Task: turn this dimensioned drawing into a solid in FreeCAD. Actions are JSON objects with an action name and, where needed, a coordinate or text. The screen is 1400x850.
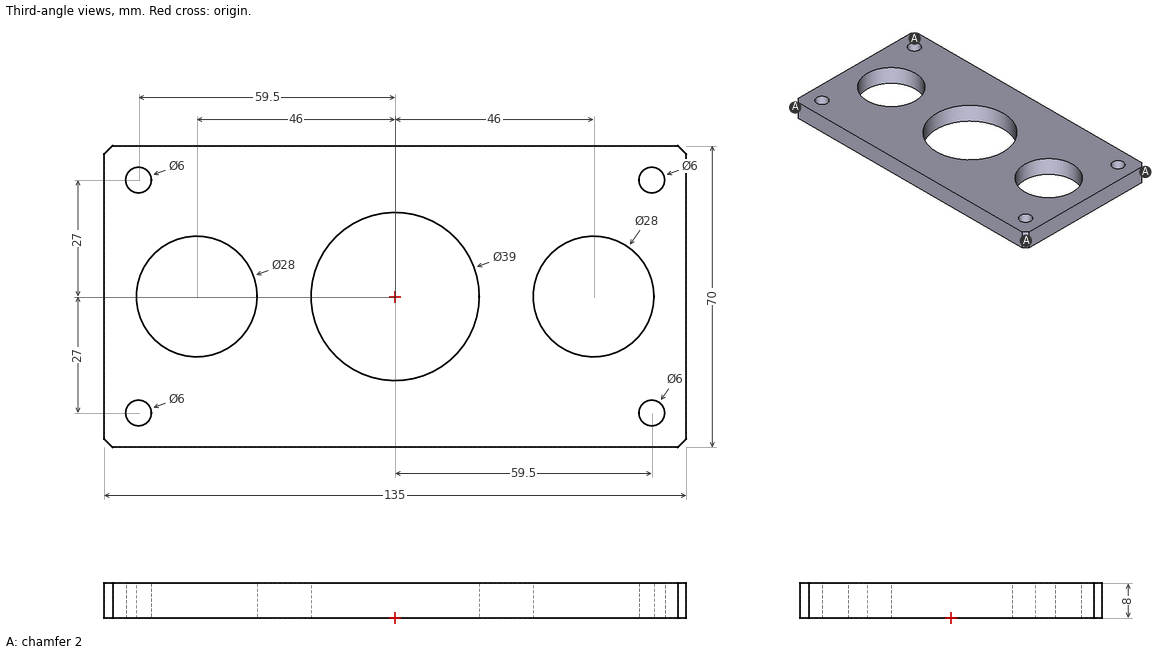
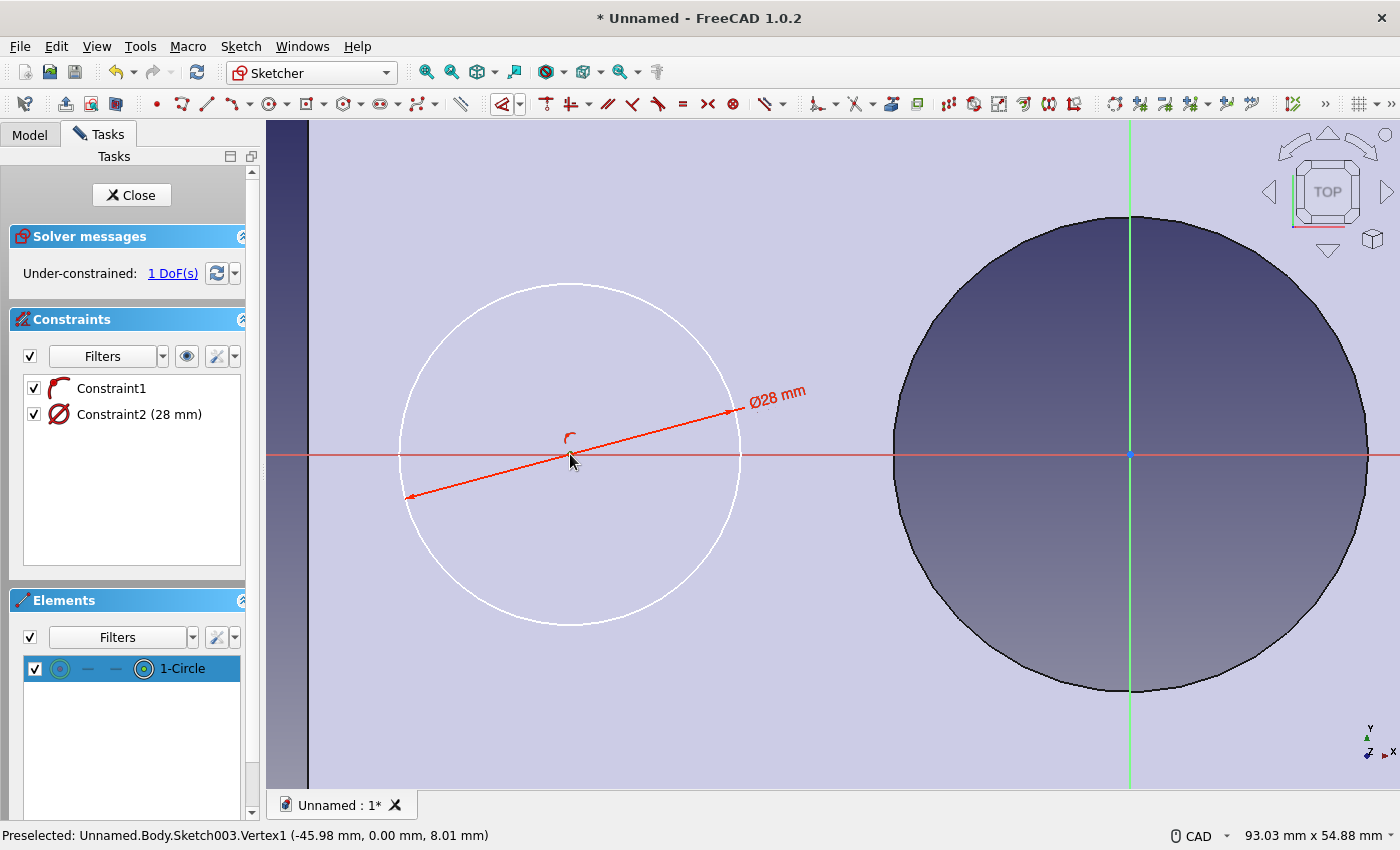
{"action": "key", "text": "l"}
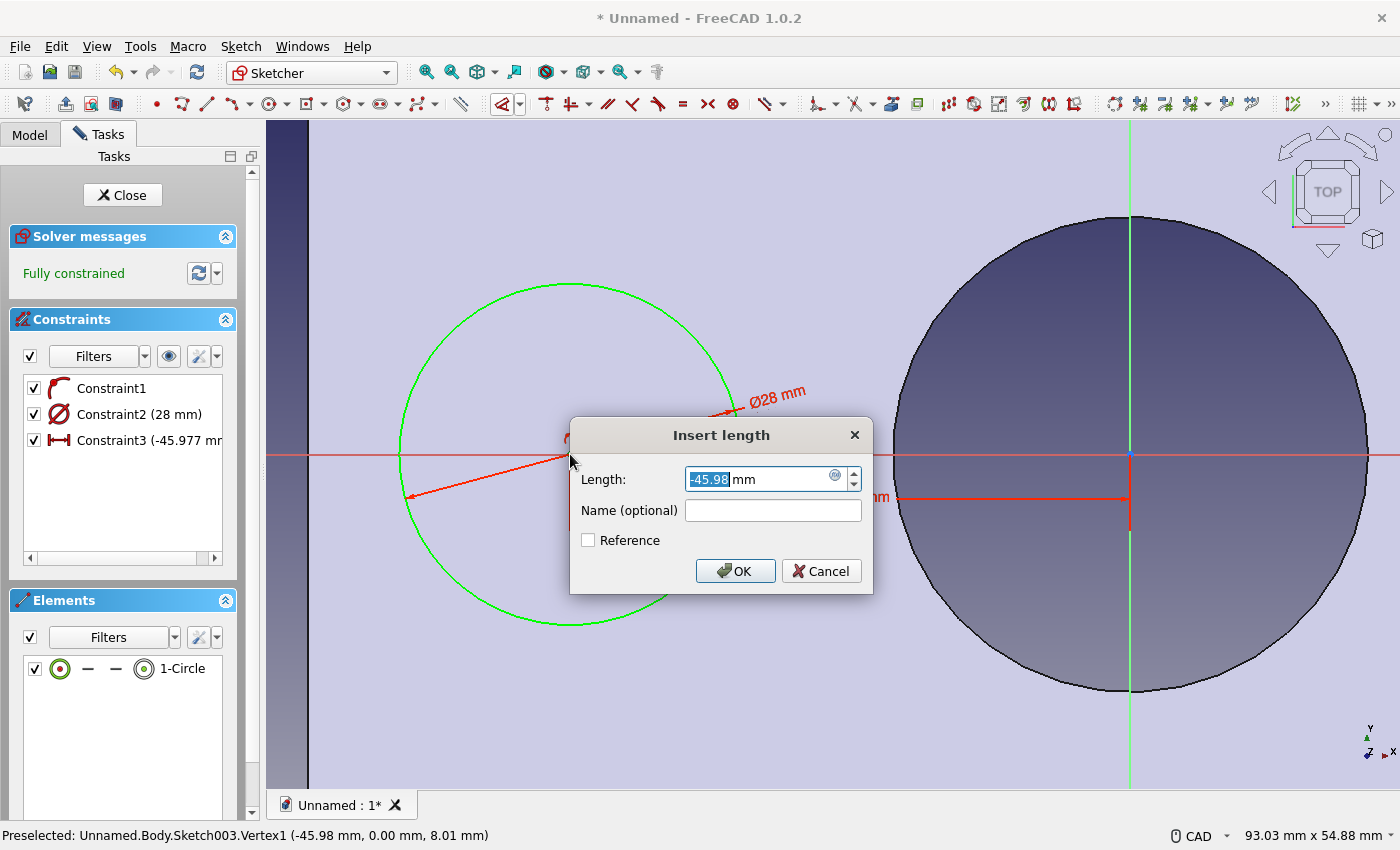
{"action": "type", "text": "-46"}
{"action": "key", "text": "Return"}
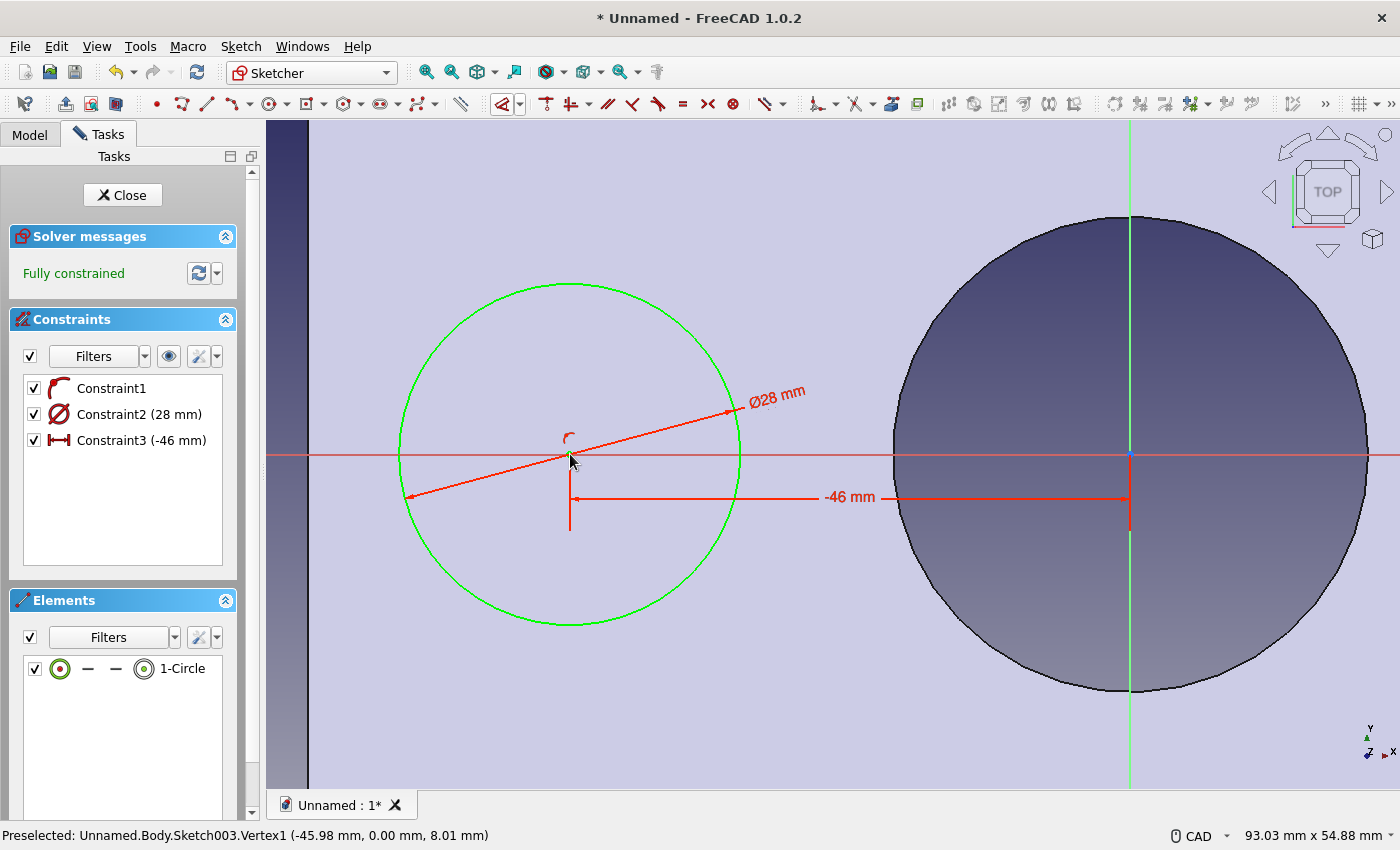
{"action": "left_click", "coordinate": [123, 195]}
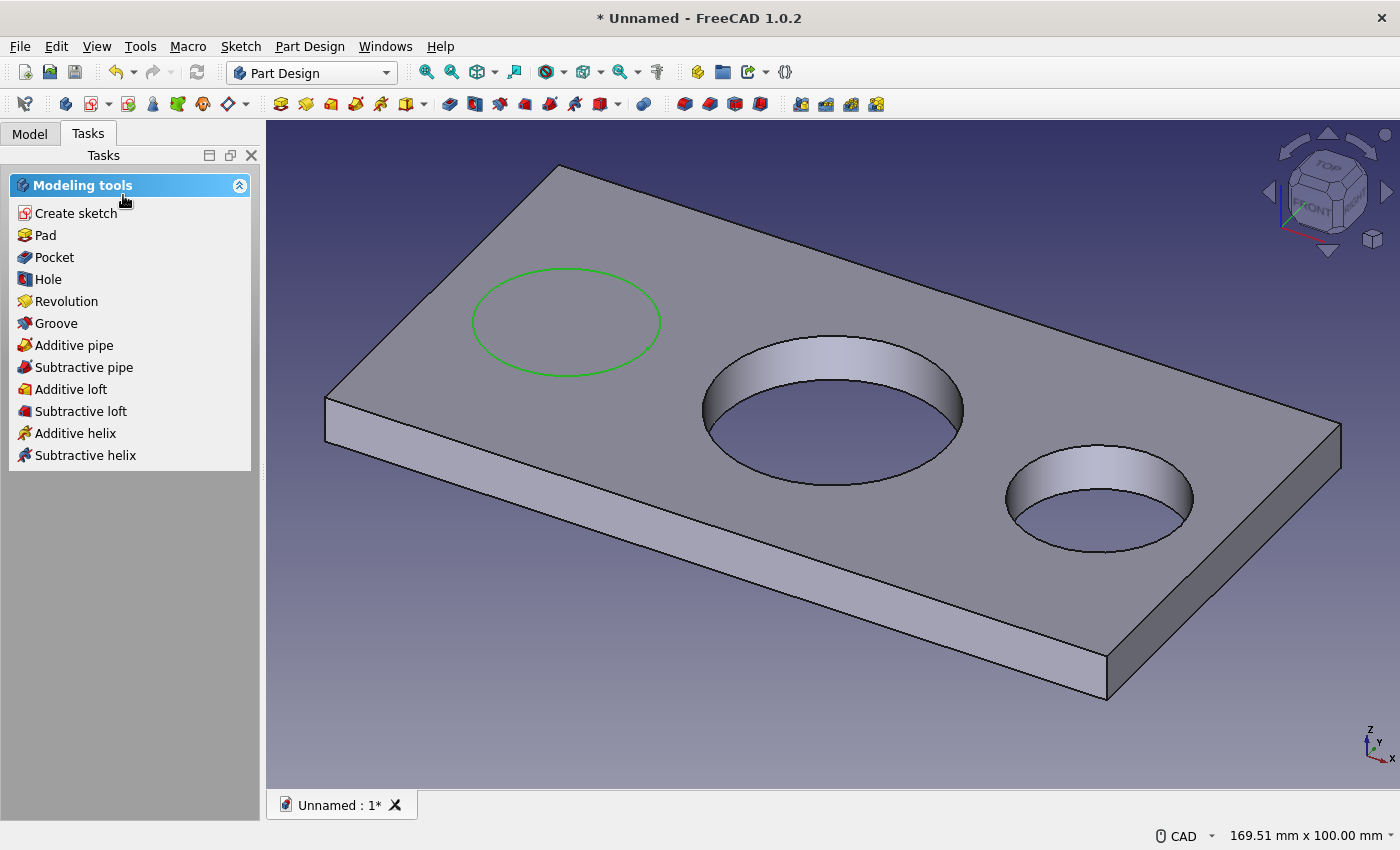
{"action": "left_click", "coordinate": [450, 104]}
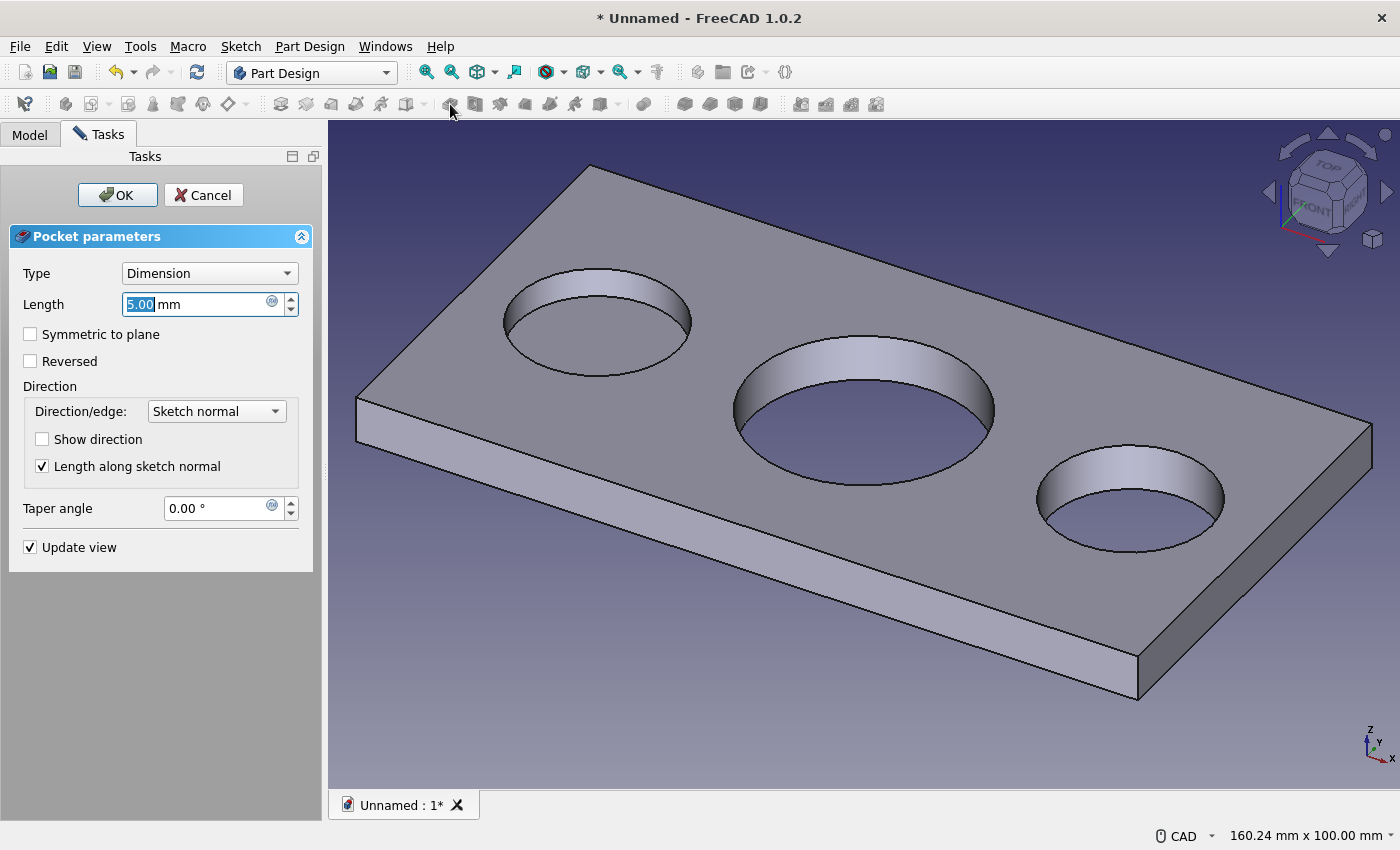
{"action": "left_click", "coordinate": [210, 274]}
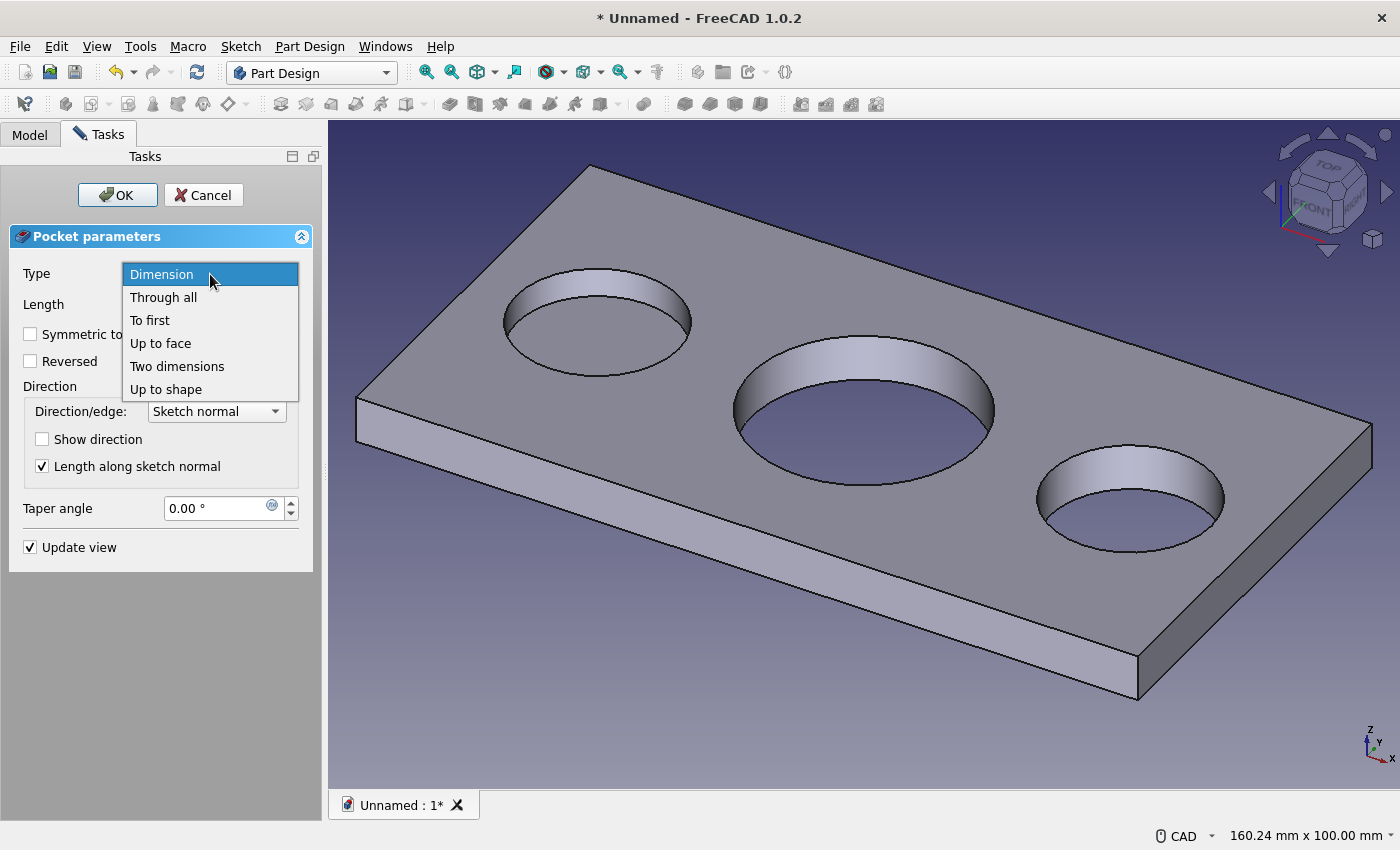
{"action": "left_click", "coordinate": [208, 320]}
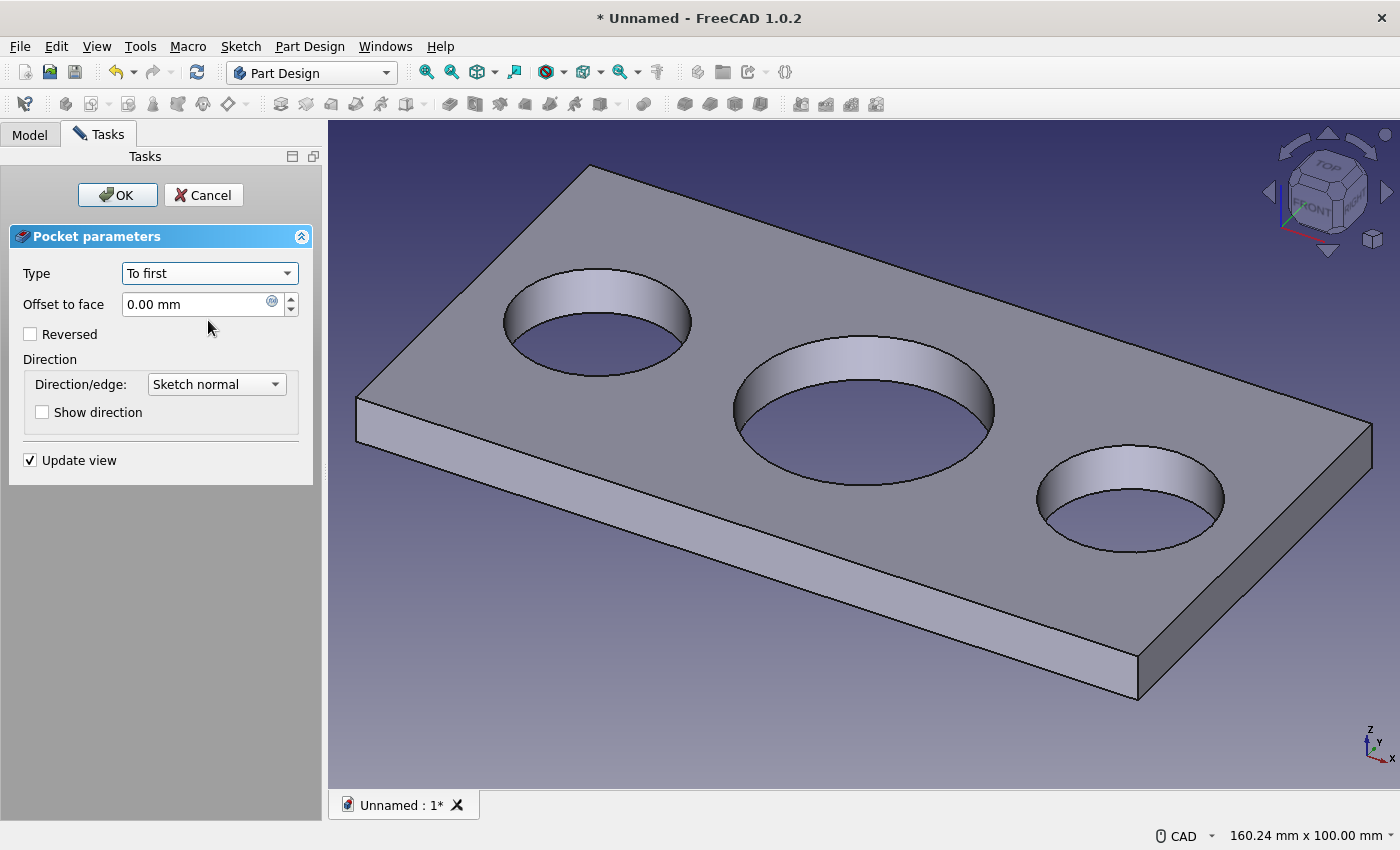
{"action": "left_click", "coordinate": [118, 195]}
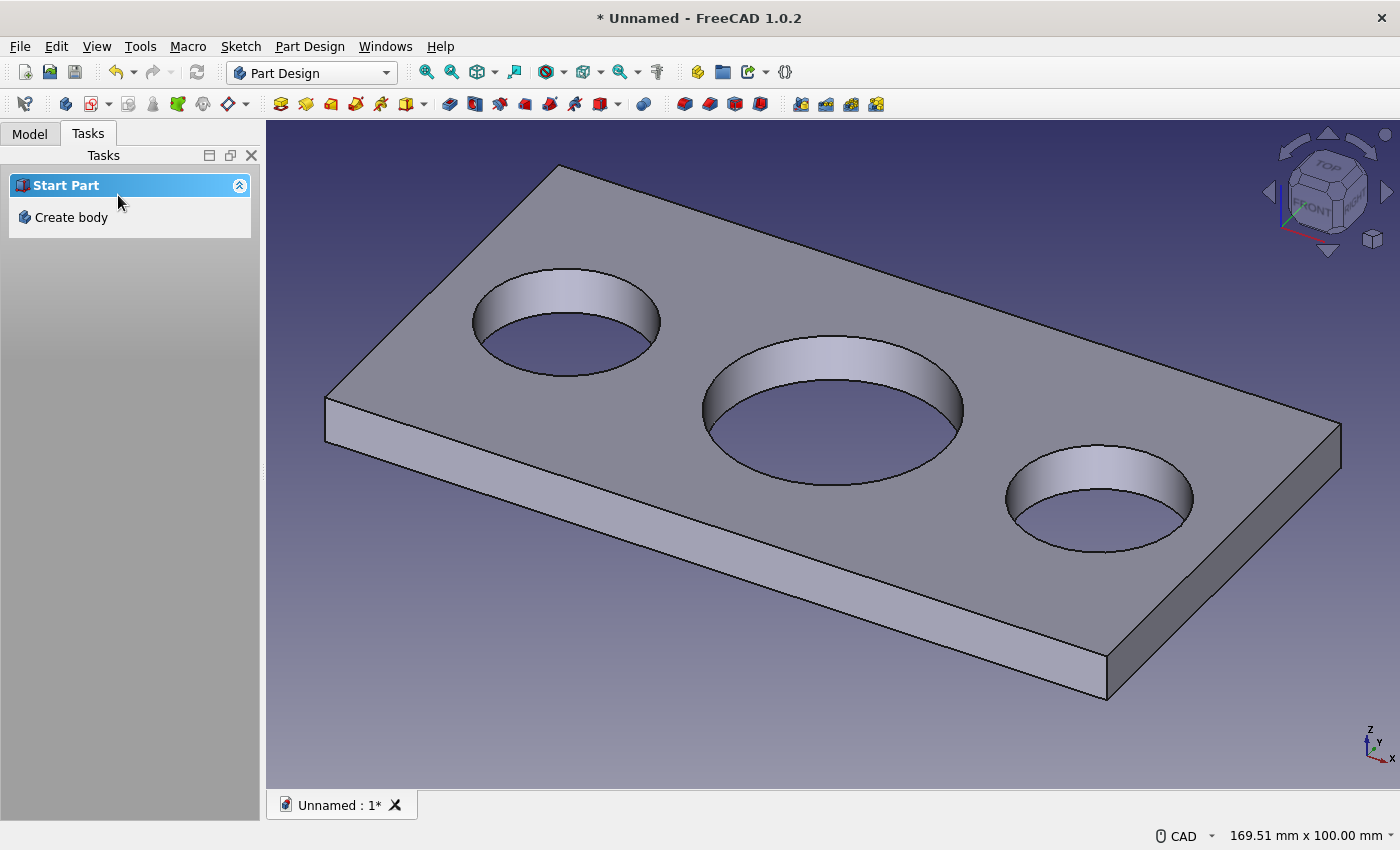
{"action": "left_click", "coordinate": [565, 232]}